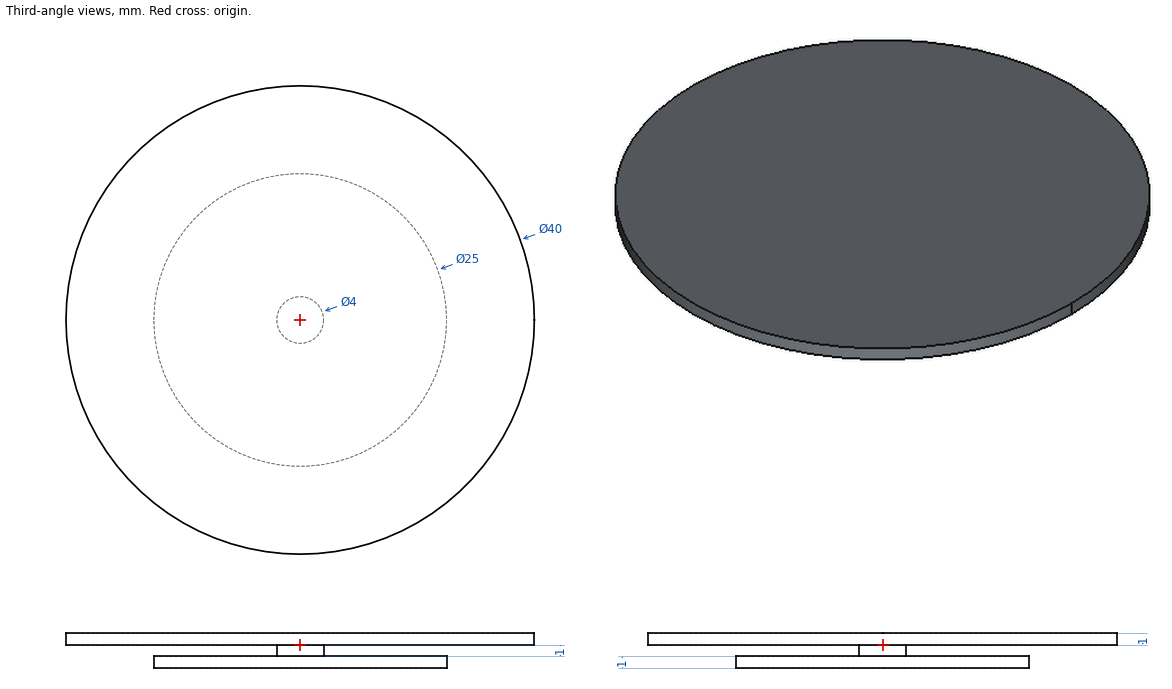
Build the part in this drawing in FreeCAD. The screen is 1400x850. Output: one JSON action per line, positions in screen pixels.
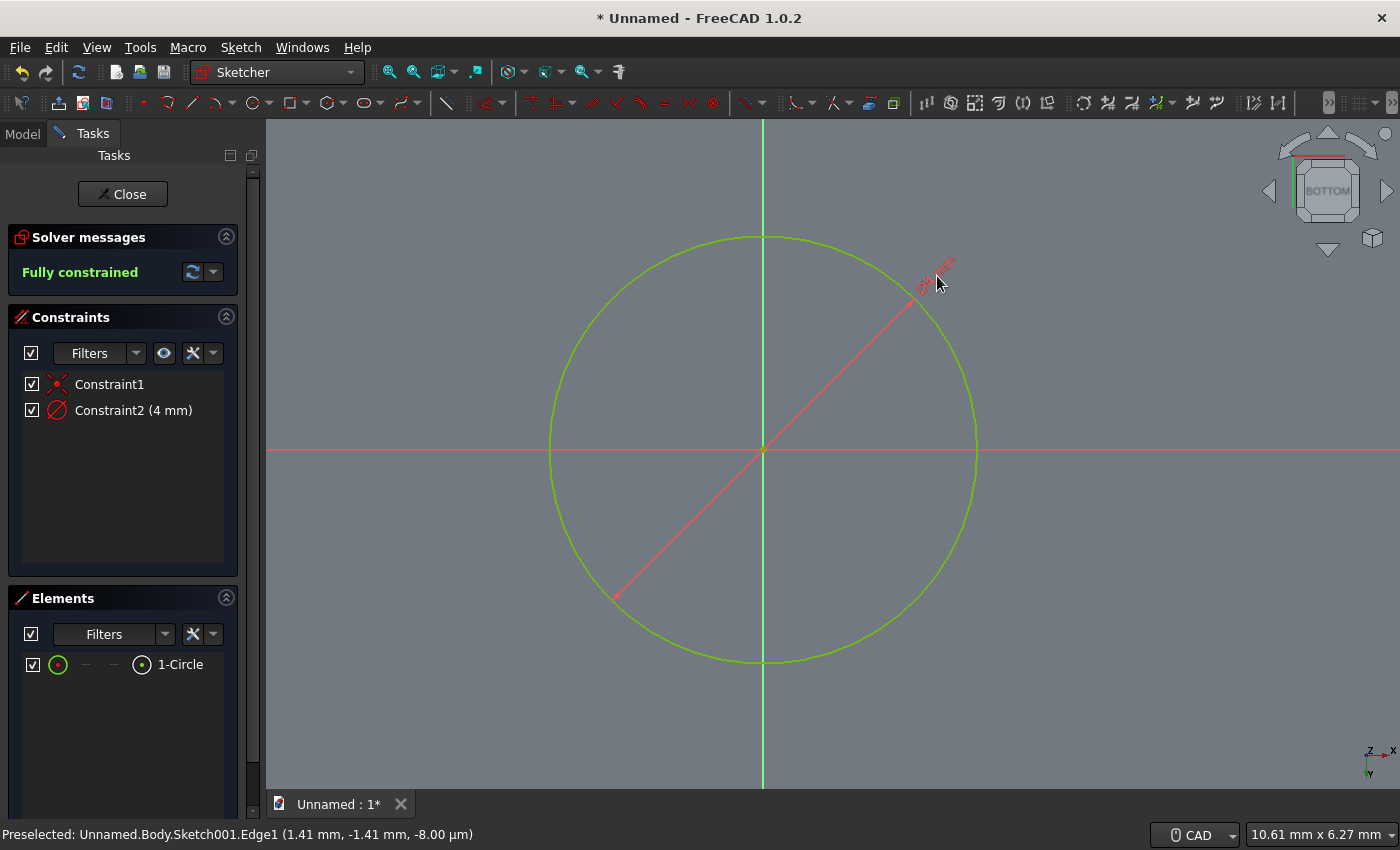
{"action": "left_click", "coordinate": [123, 194]}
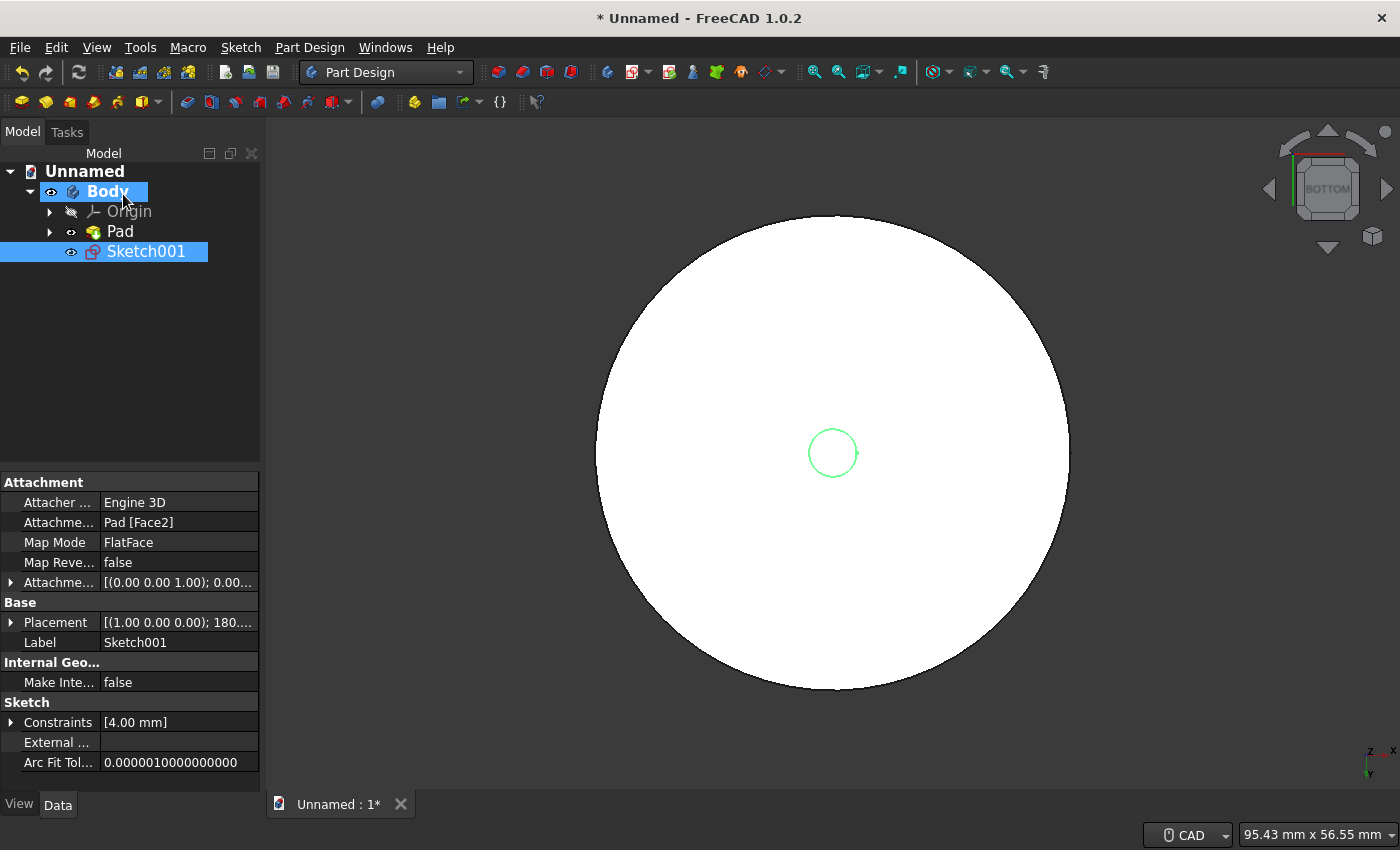
{"action": "left_click", "coordinate": [22, 102]}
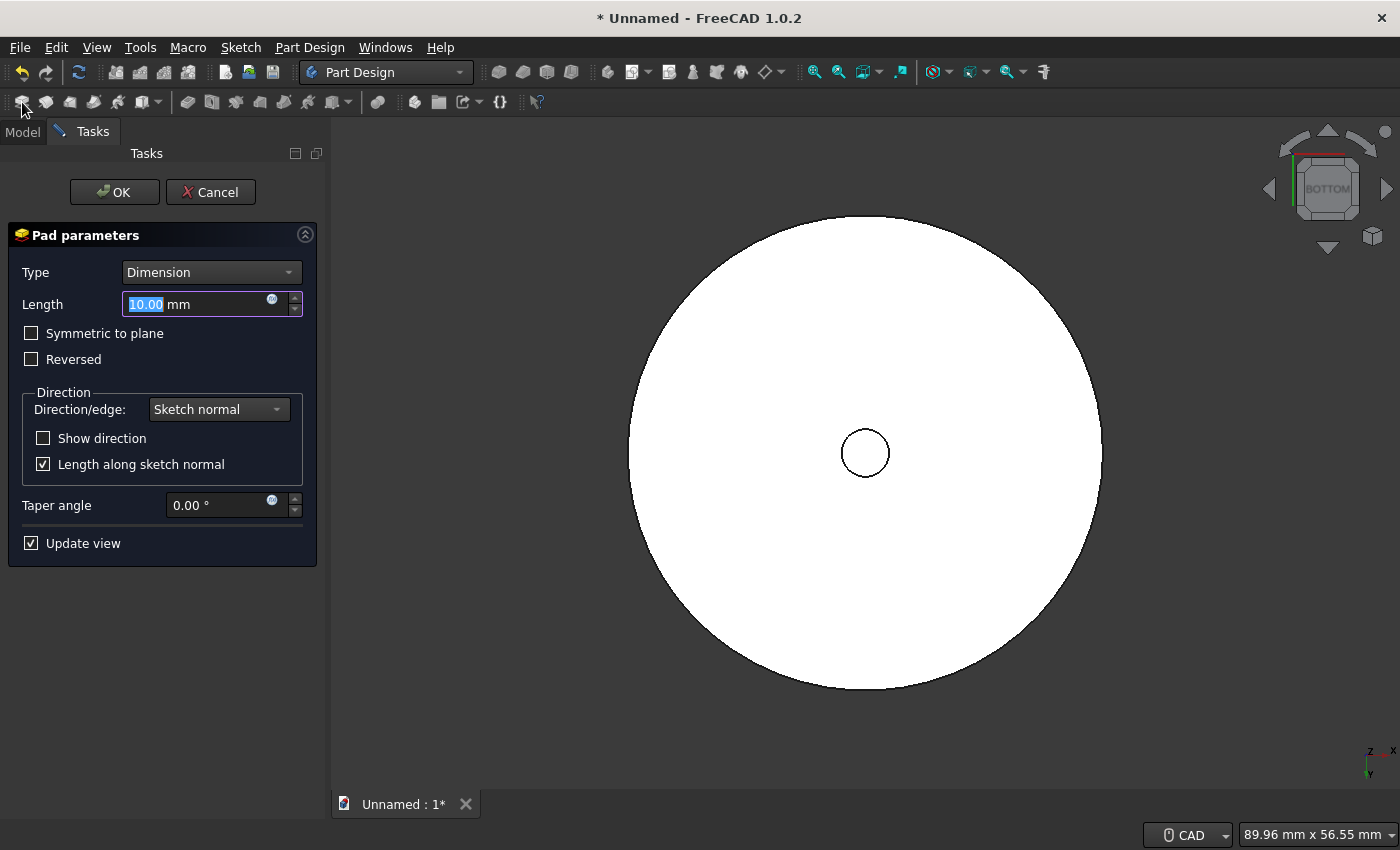
{"action": "type", "text": "1"}
{"action": "key", "text": "Tab"}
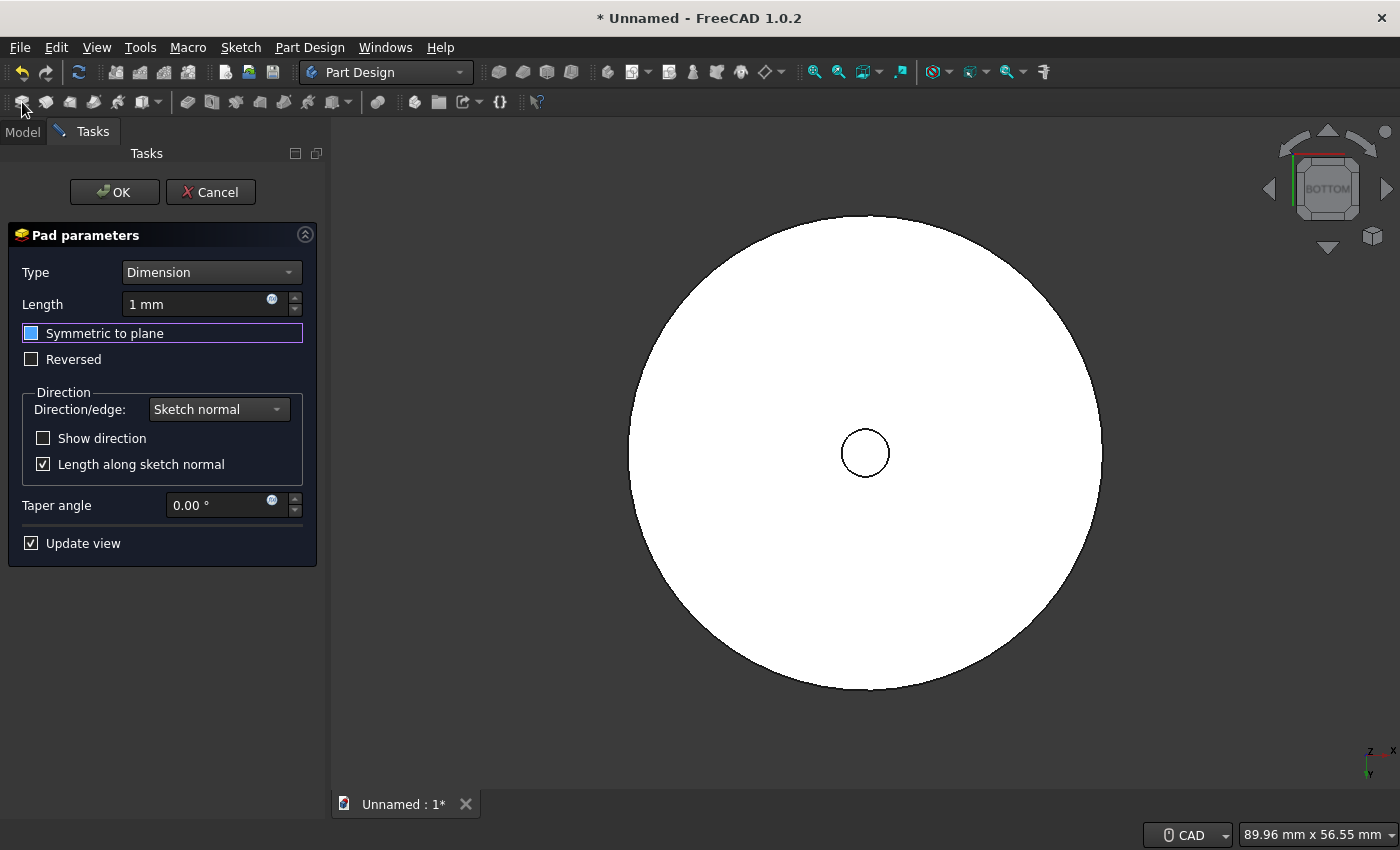
{"action": "left_click", "coordinate": [115, 192]}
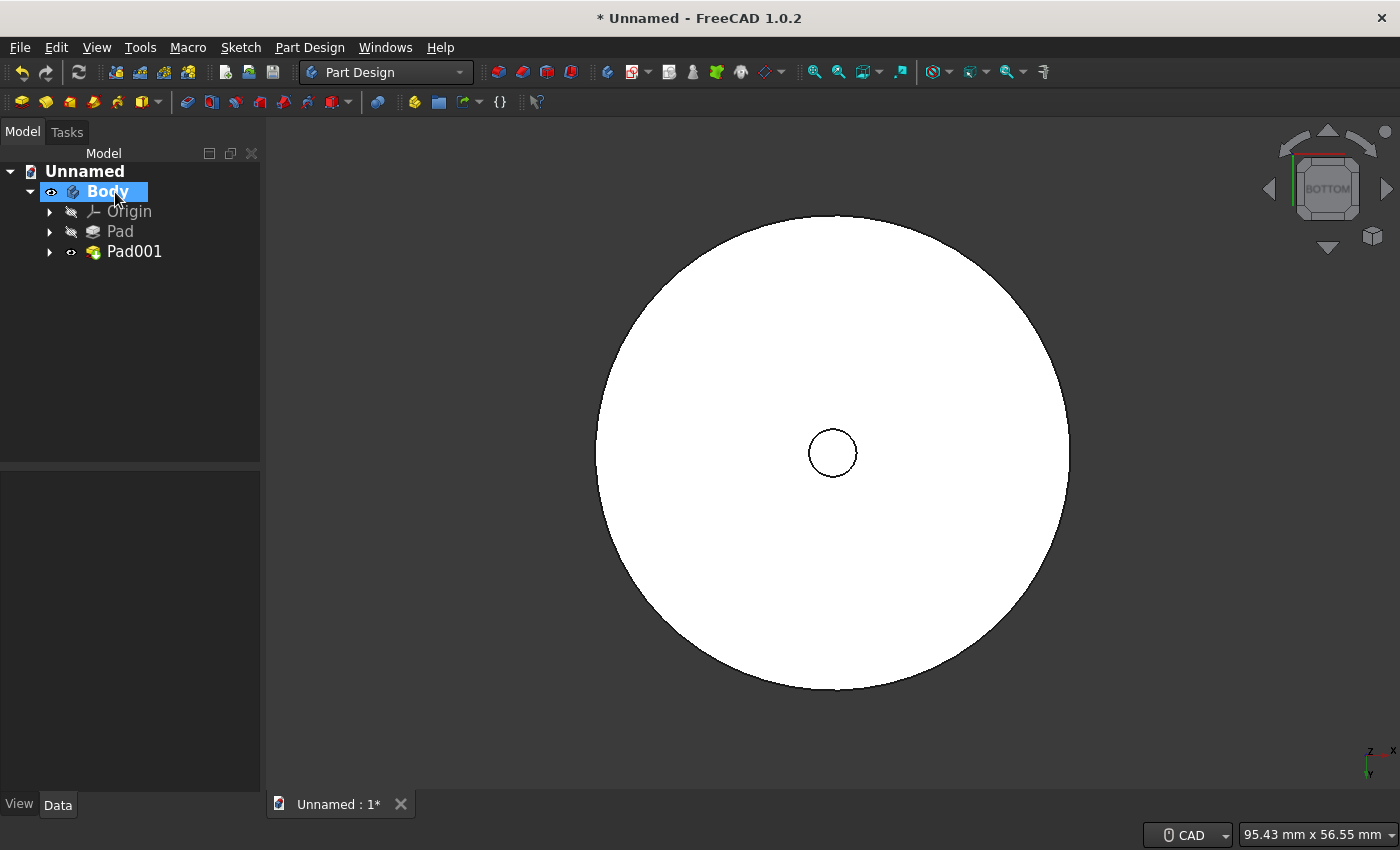
{"action": "left_click", "coordinate": [833, 452]}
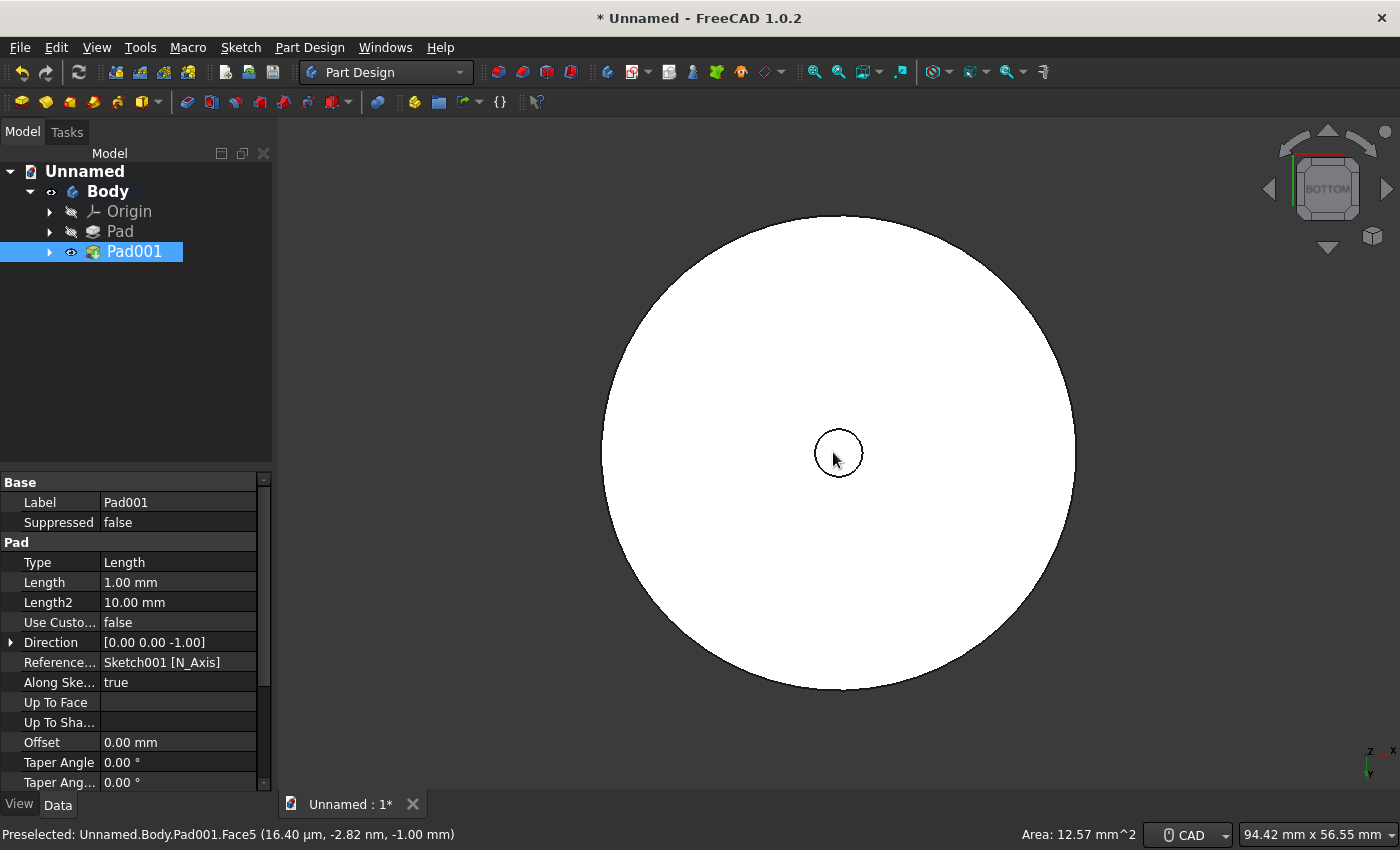
{"action": "left_click", "coordinate": [632, 72]}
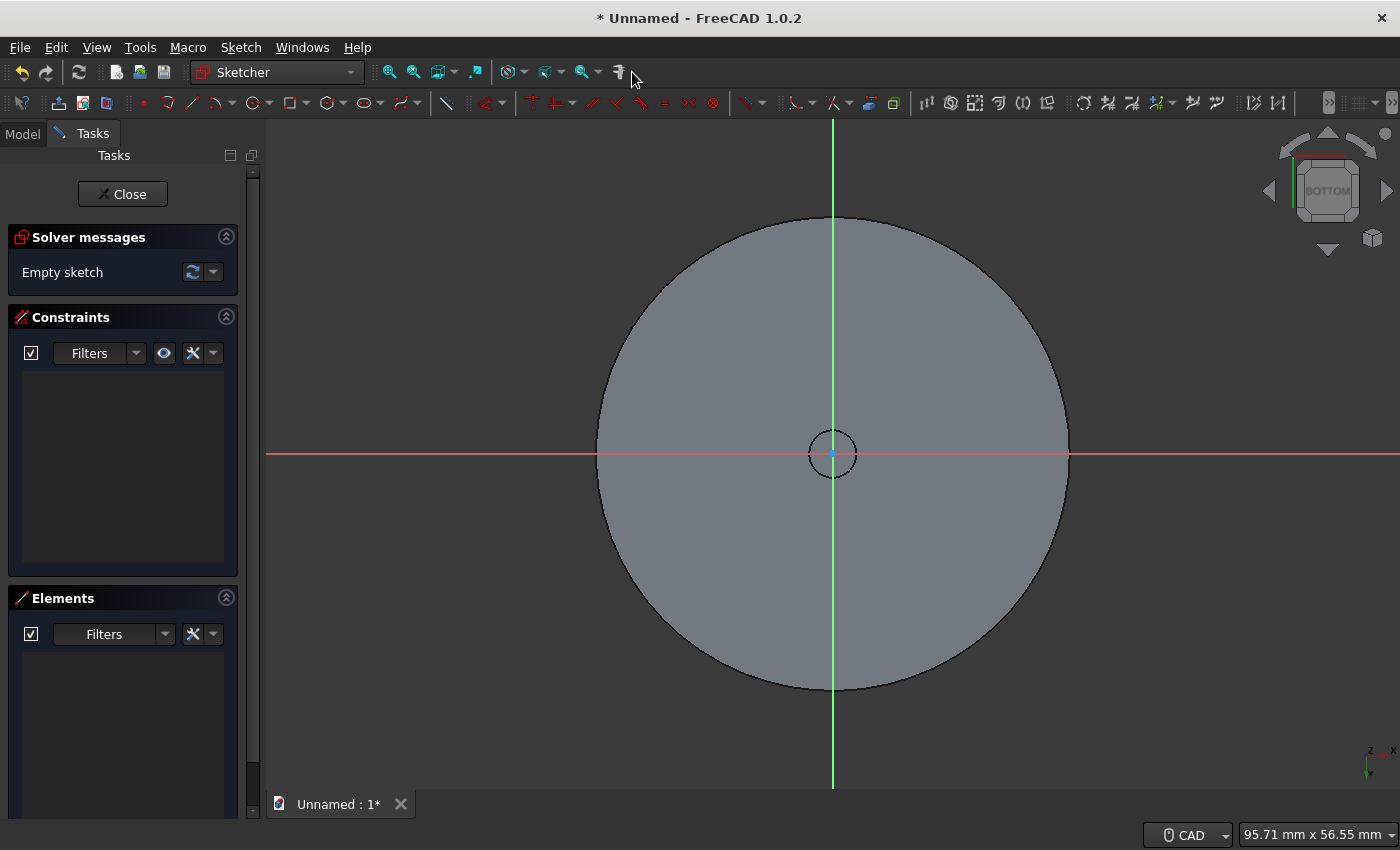
{"action": "scroll", "coordinate": [972, 454], "scroll_direction": "up", "scroll_amount": 2}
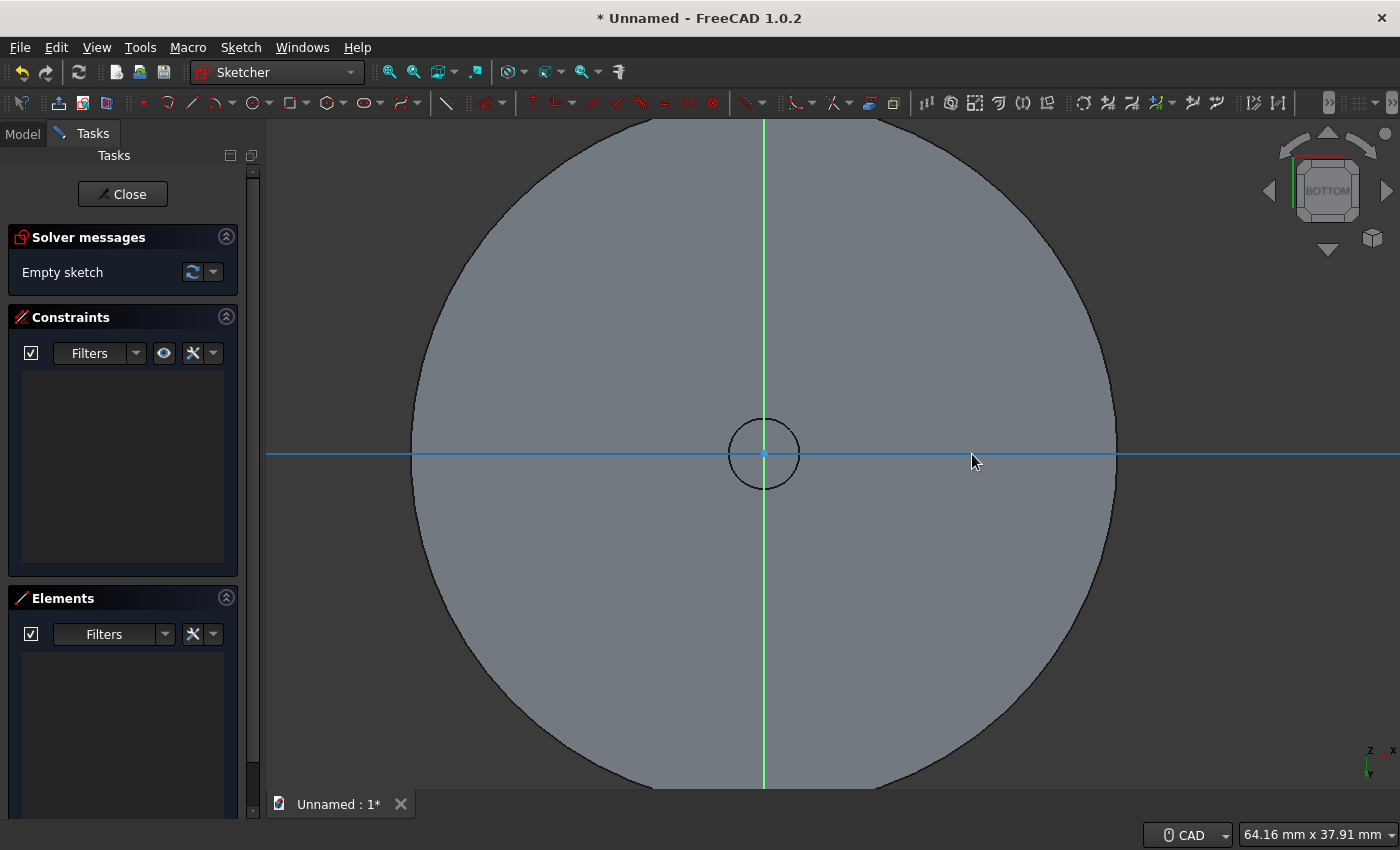
{"action": "key", "text": "g c"}